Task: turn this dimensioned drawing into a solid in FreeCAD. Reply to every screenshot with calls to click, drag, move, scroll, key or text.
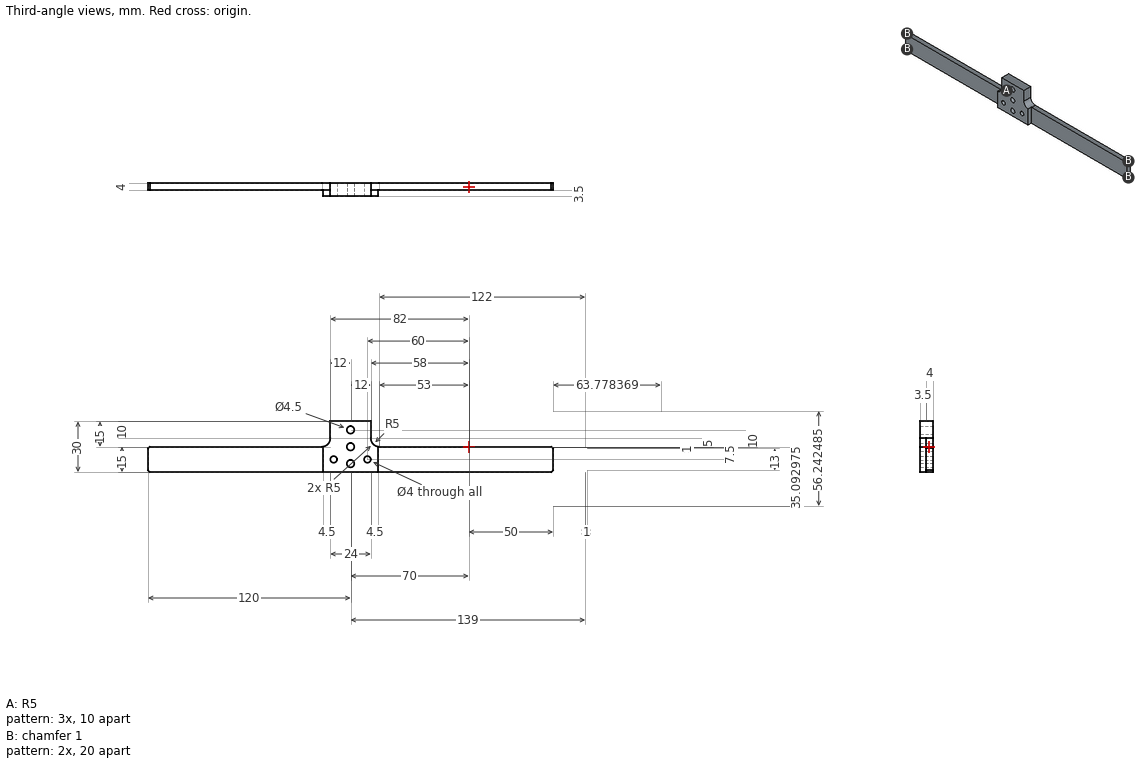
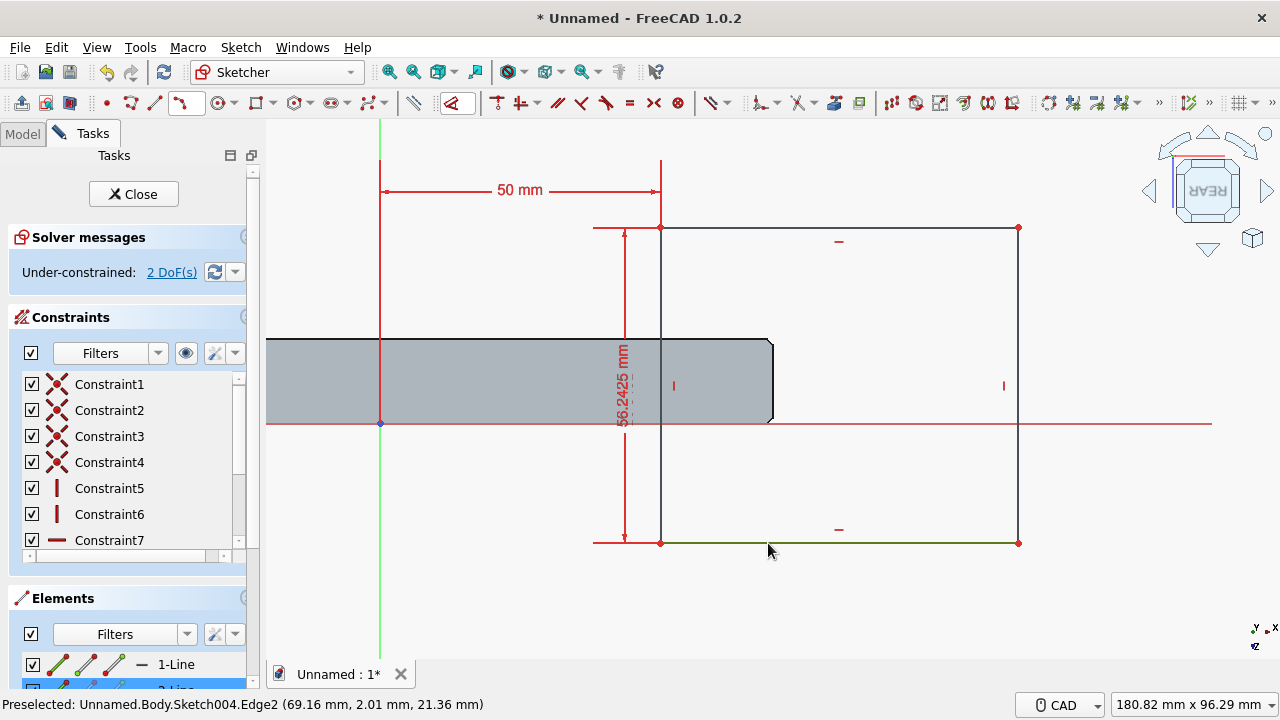
click(470, 104)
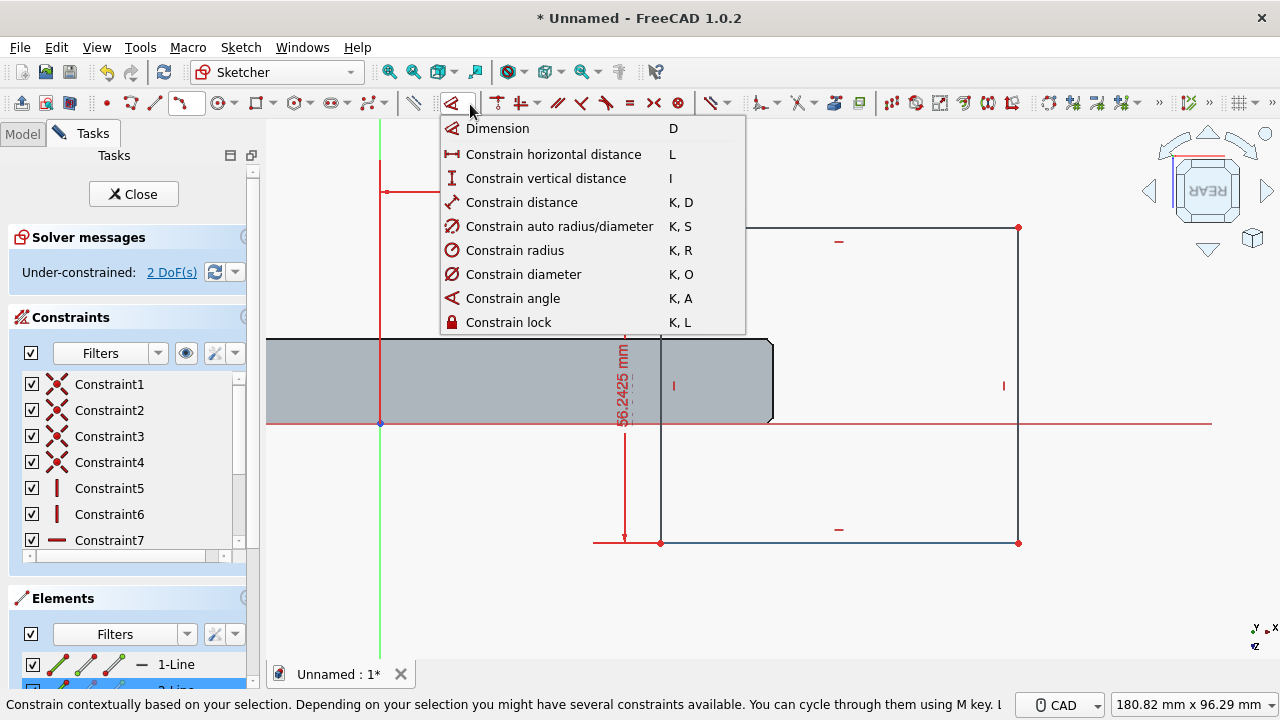
click(593, 154)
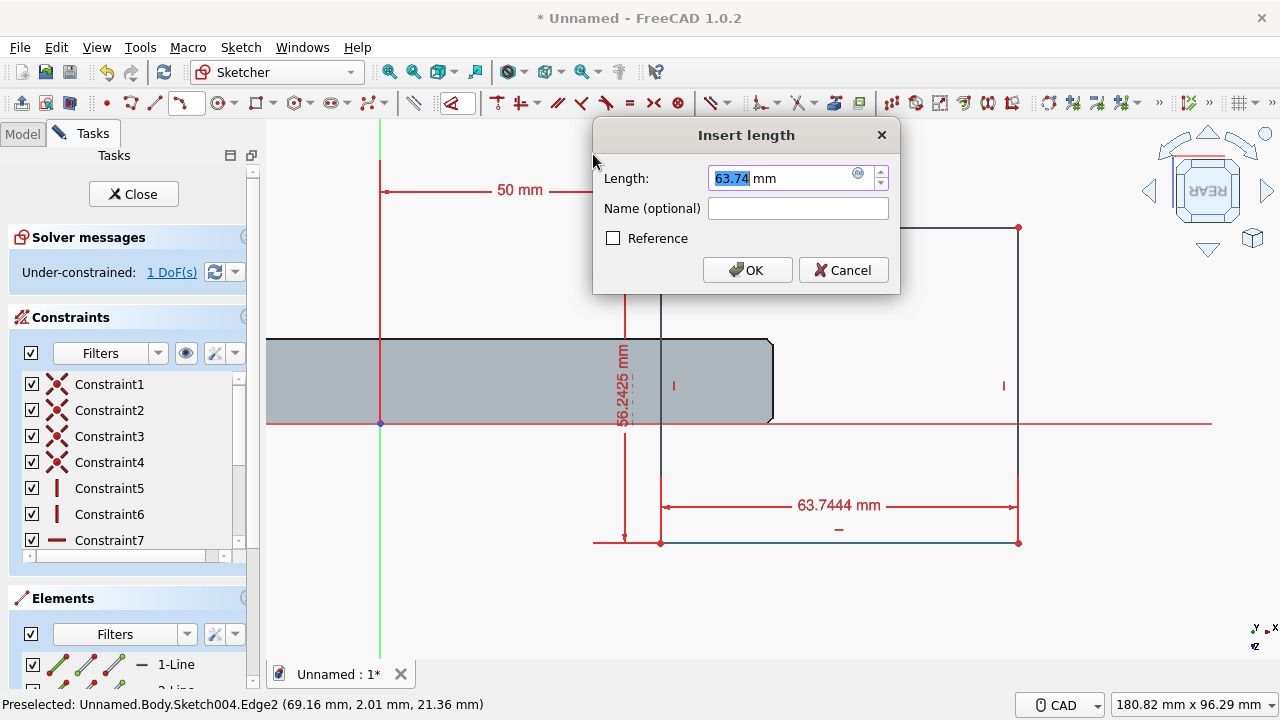
text(63.778369)
key(Return)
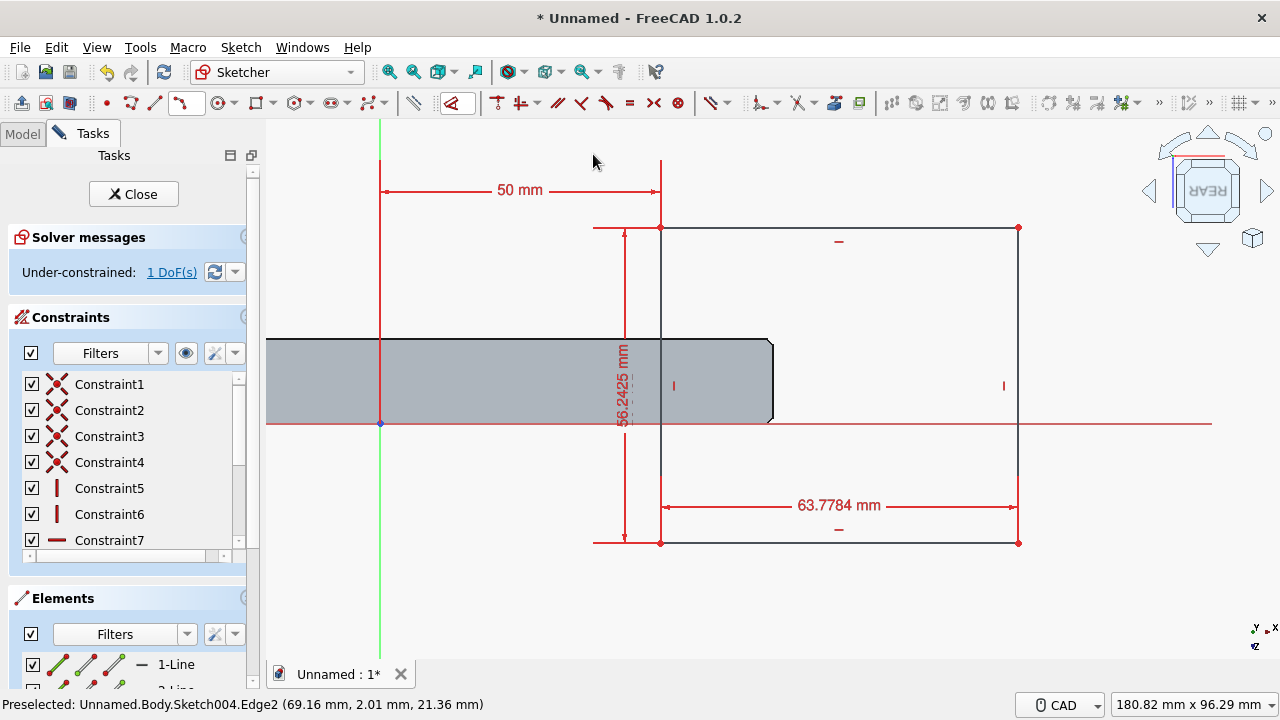
click(661, 228)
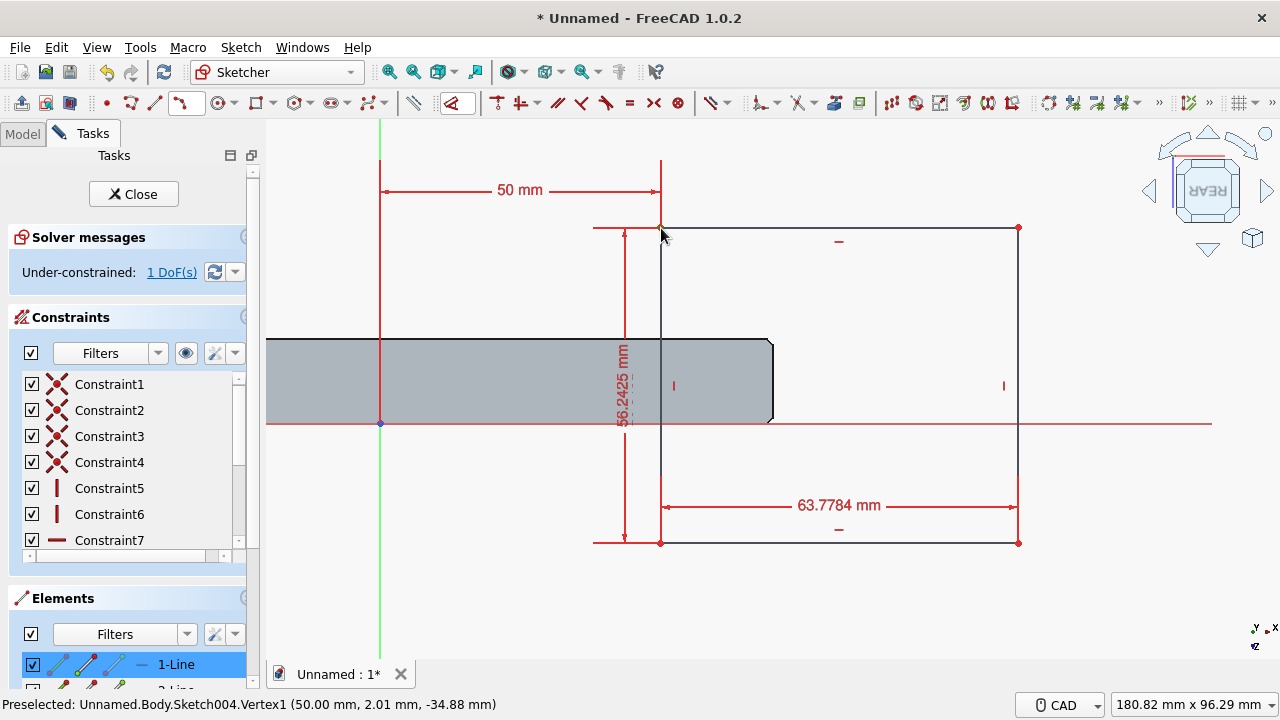
click(470, 104)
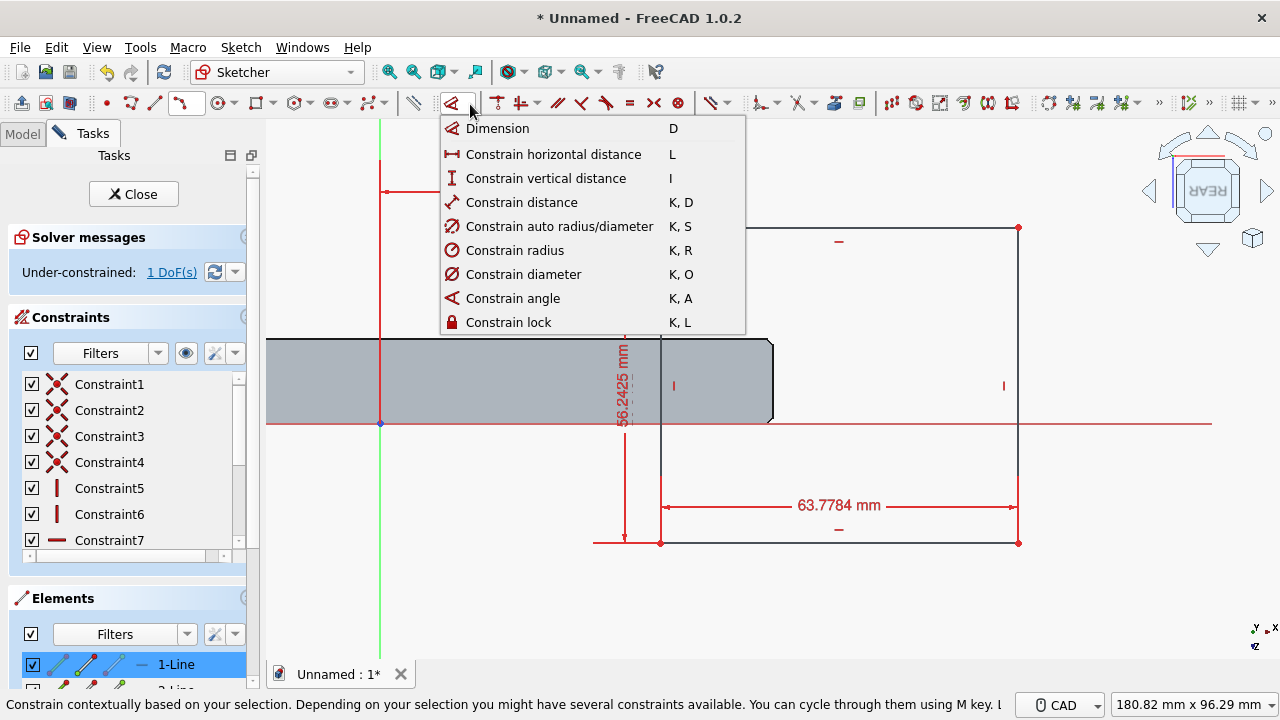
click(593, 178)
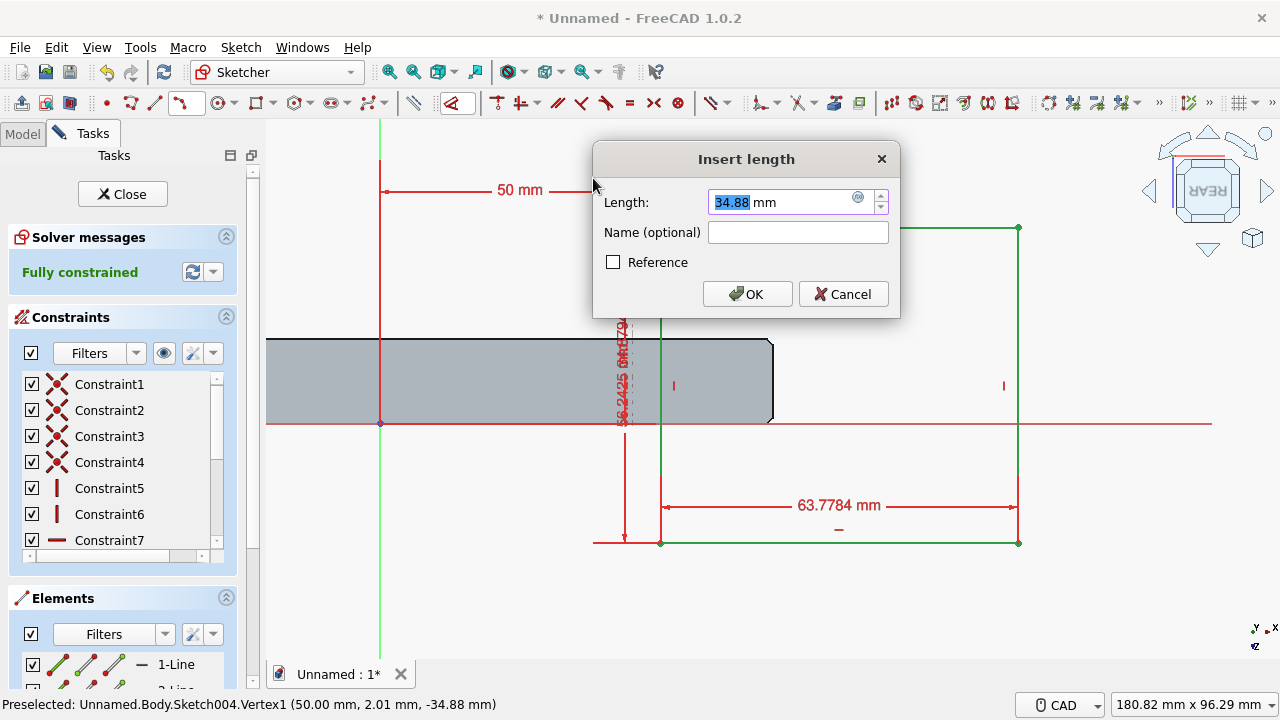
text(35.092975)
key(Return)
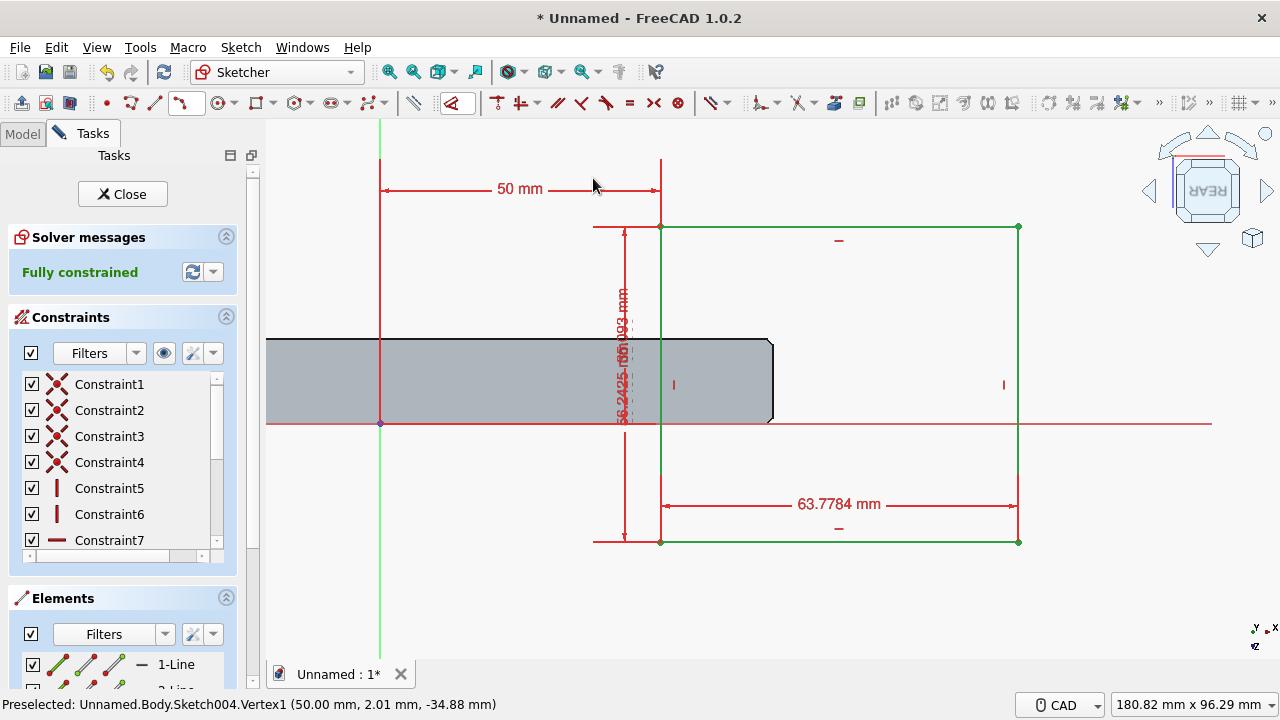
click(123, 194)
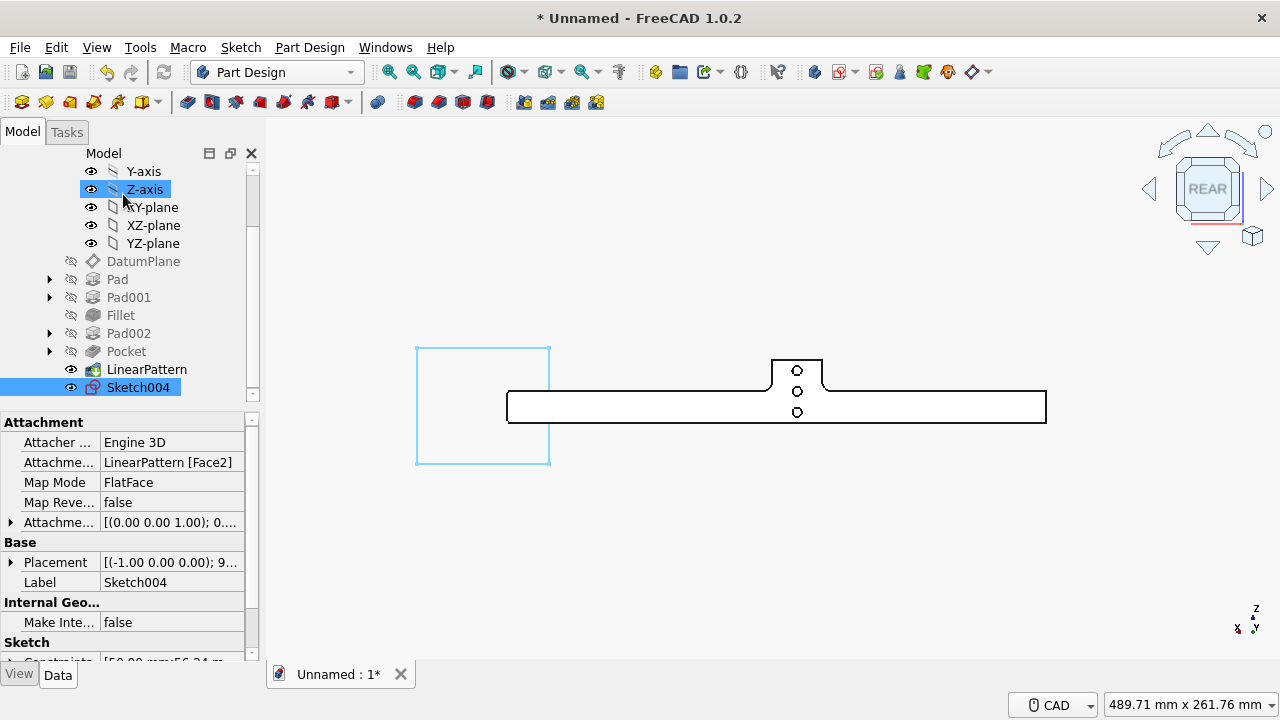
click(188, 102)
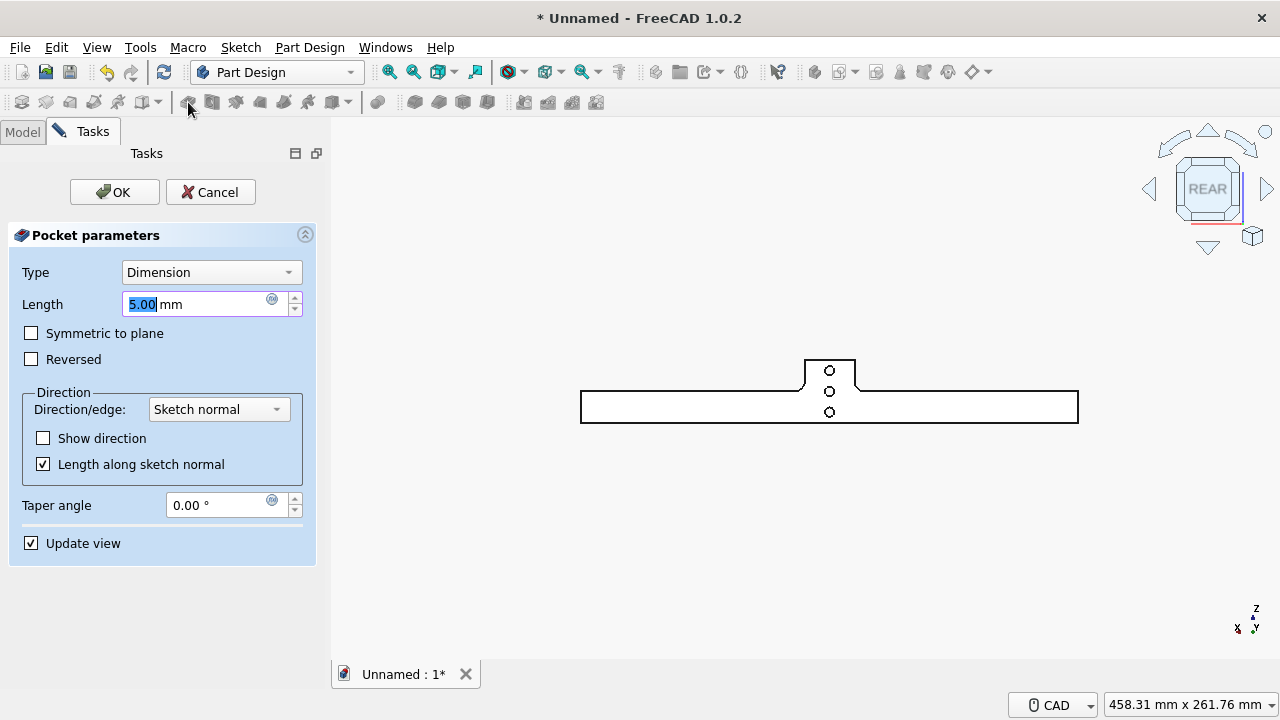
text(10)
key(Tab)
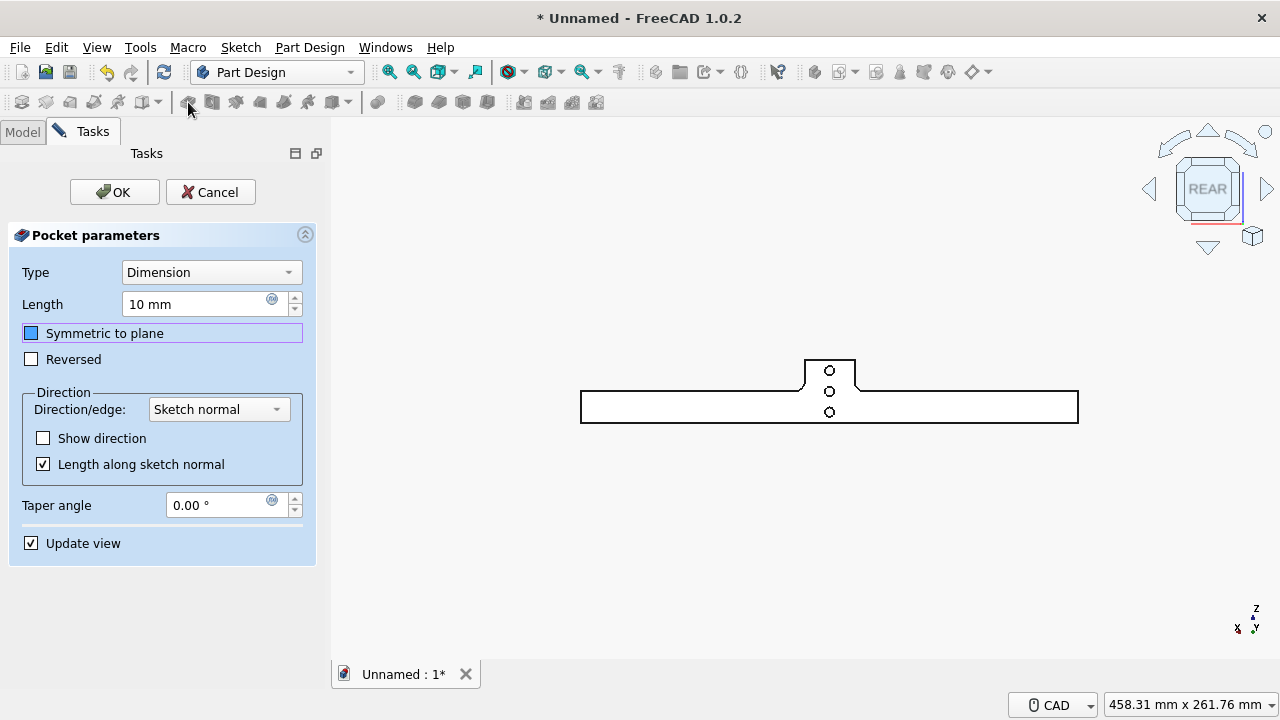
click(115, 192)